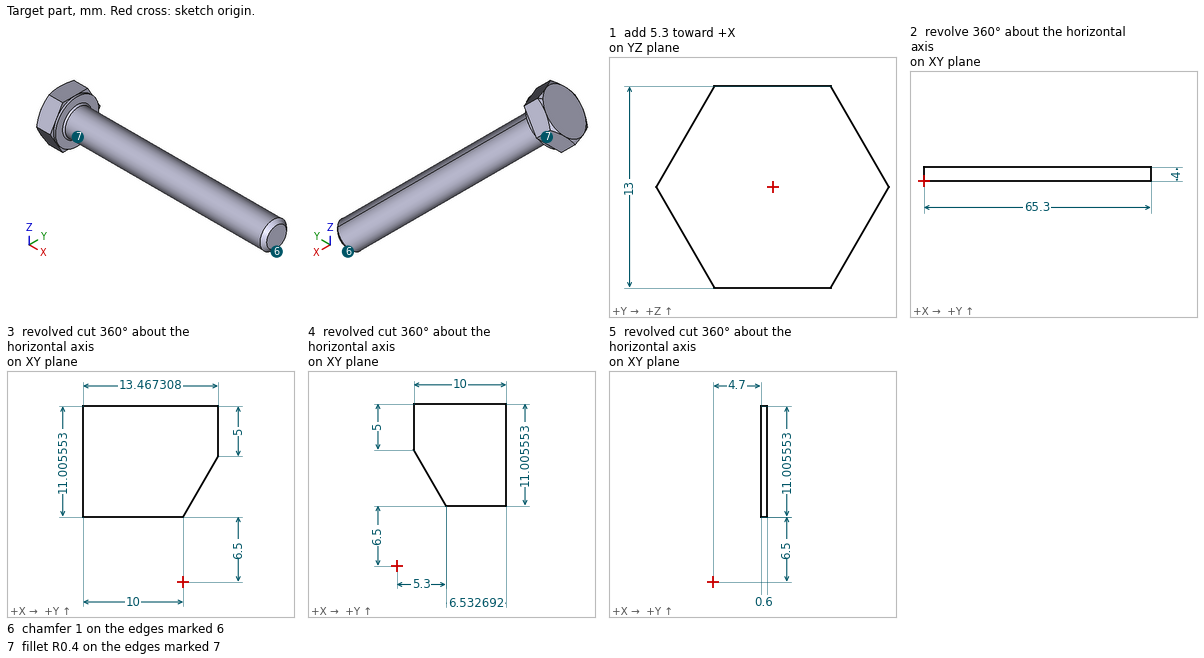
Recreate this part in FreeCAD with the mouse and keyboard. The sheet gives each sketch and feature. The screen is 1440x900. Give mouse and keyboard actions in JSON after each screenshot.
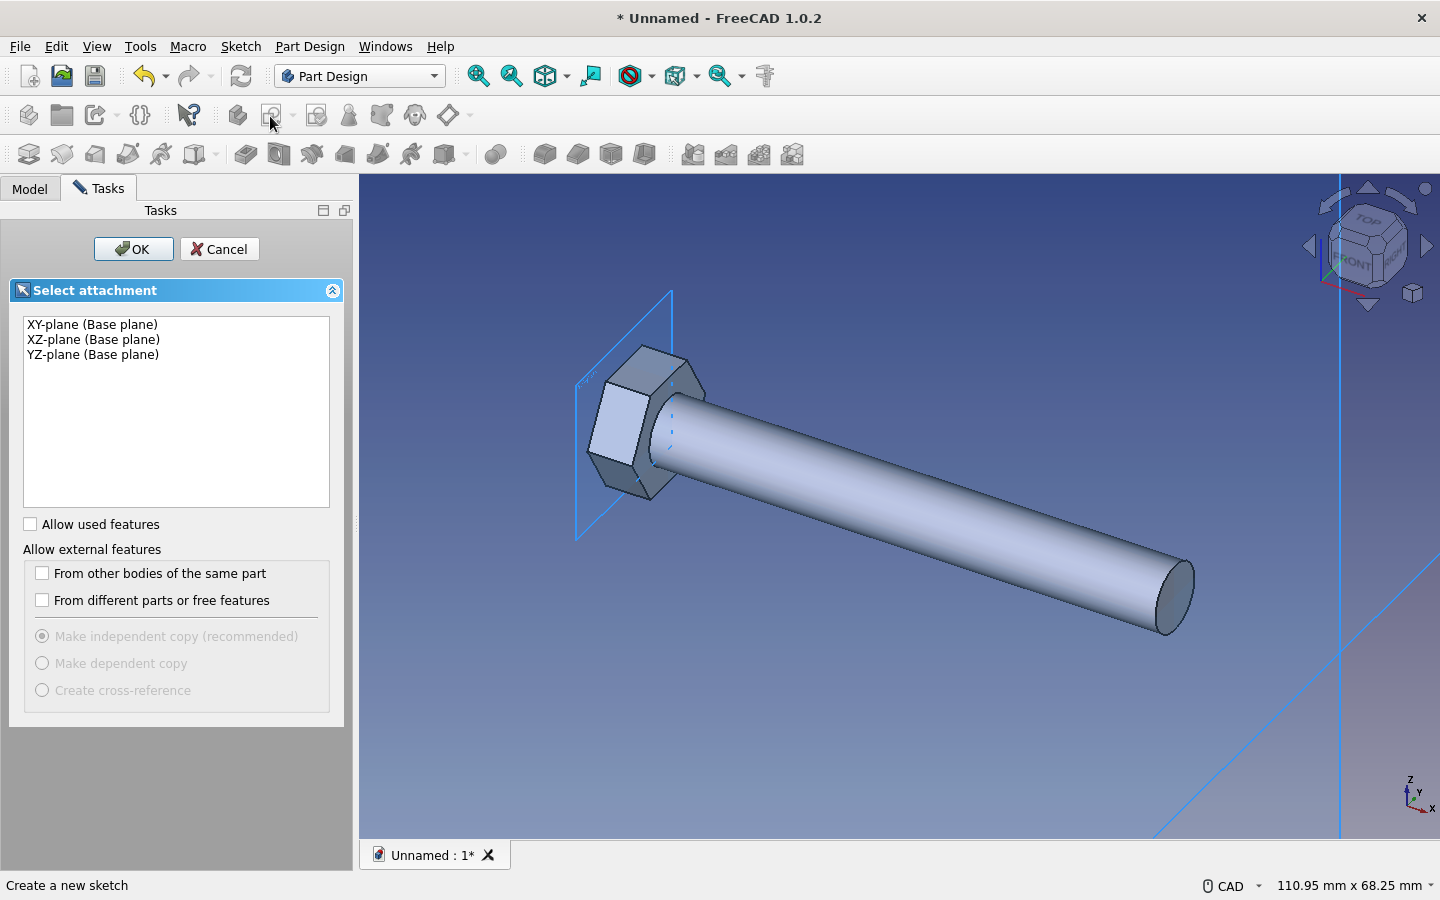
{"action": "left_click", "coordinate": [84, 324]}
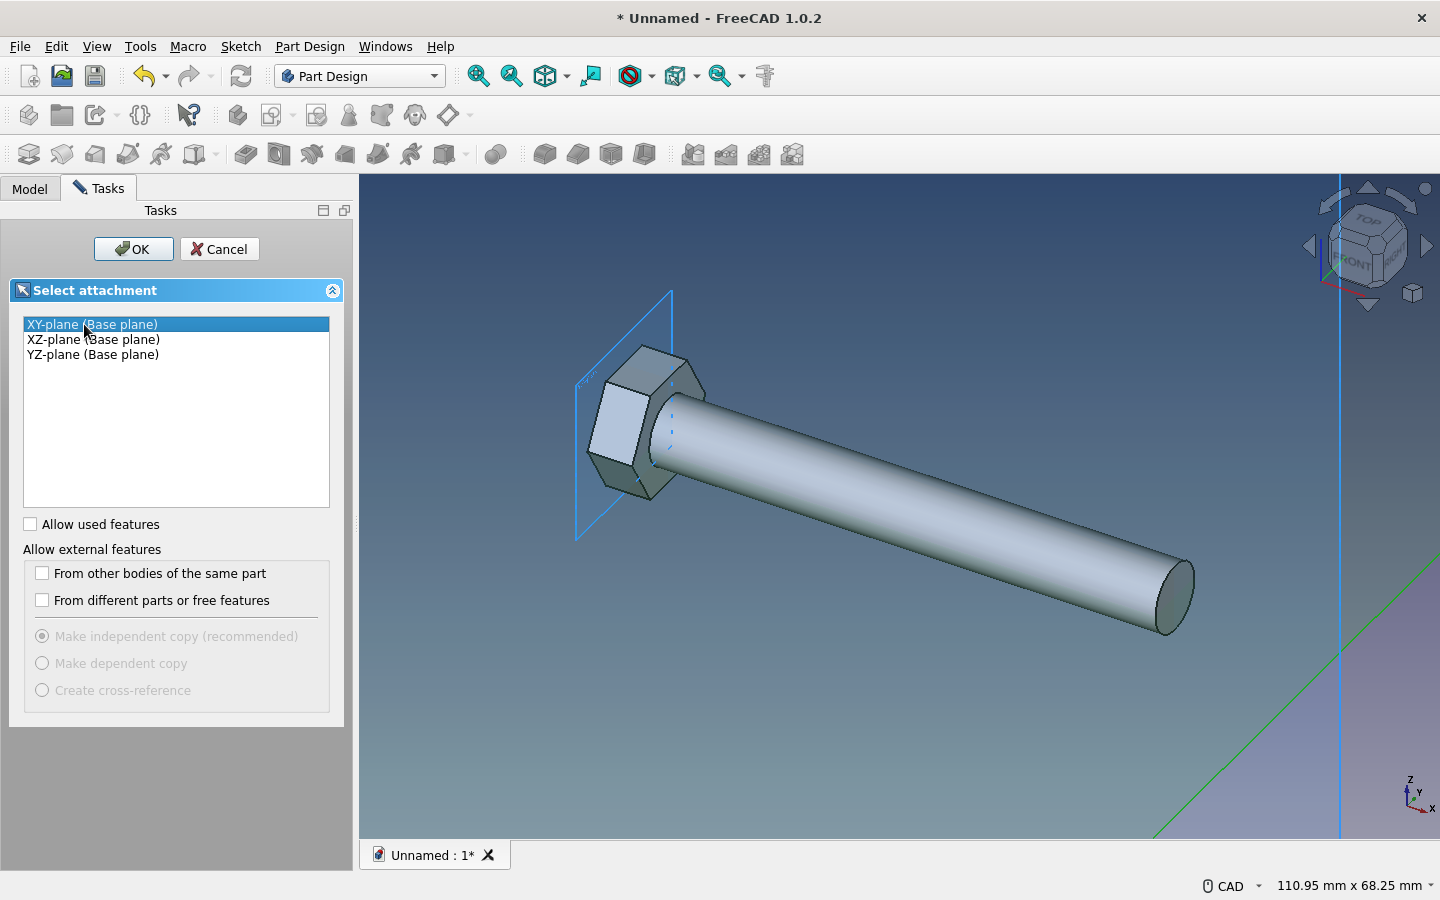
{"action": "left_click", "coordinate": [134, 249]}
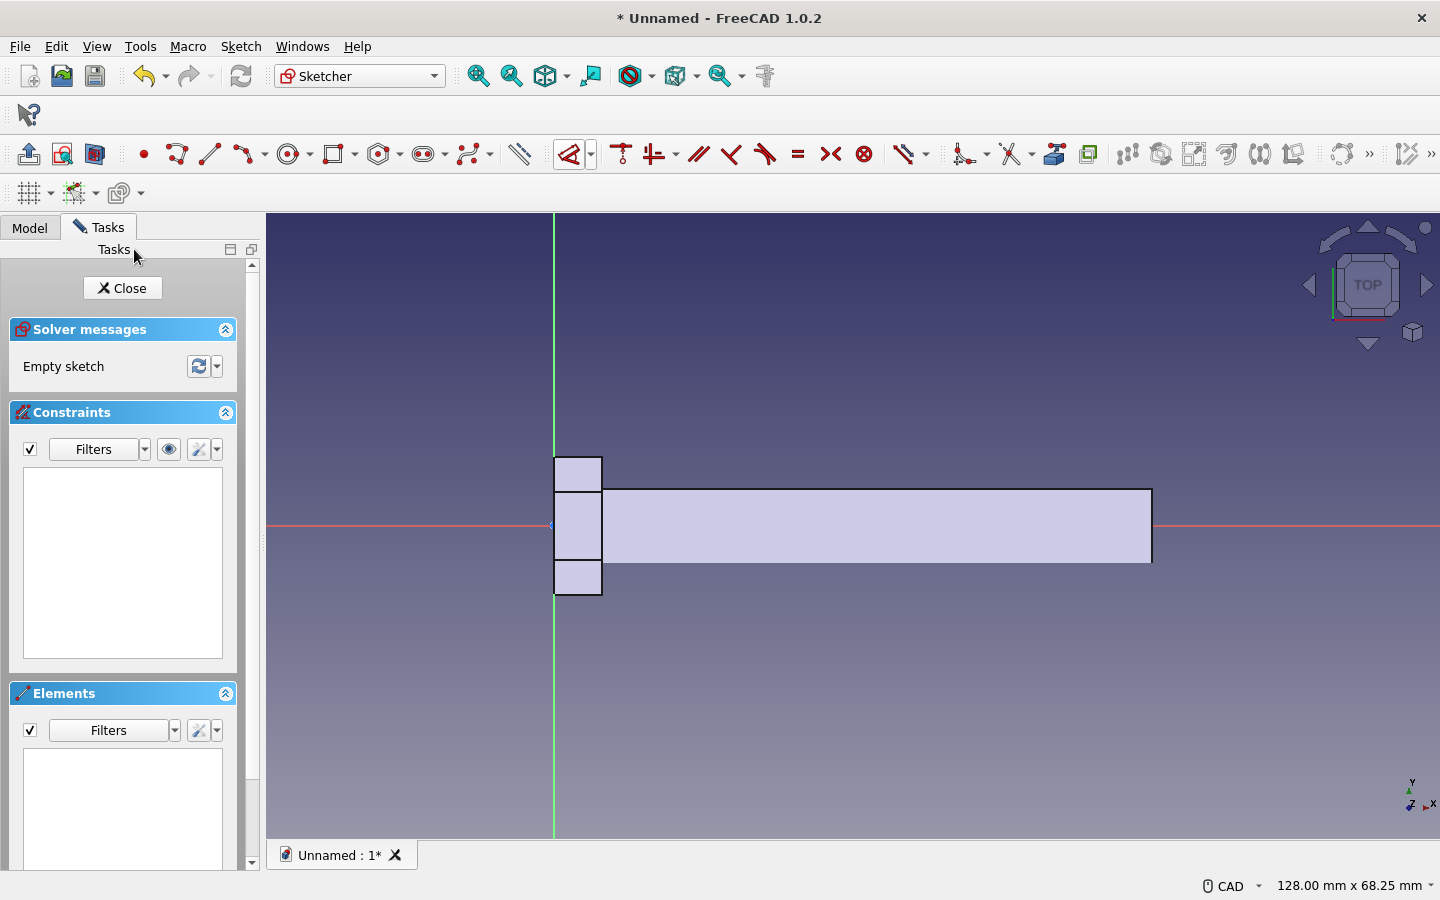
{"action": "left_click", "coordinate": [95, 154]}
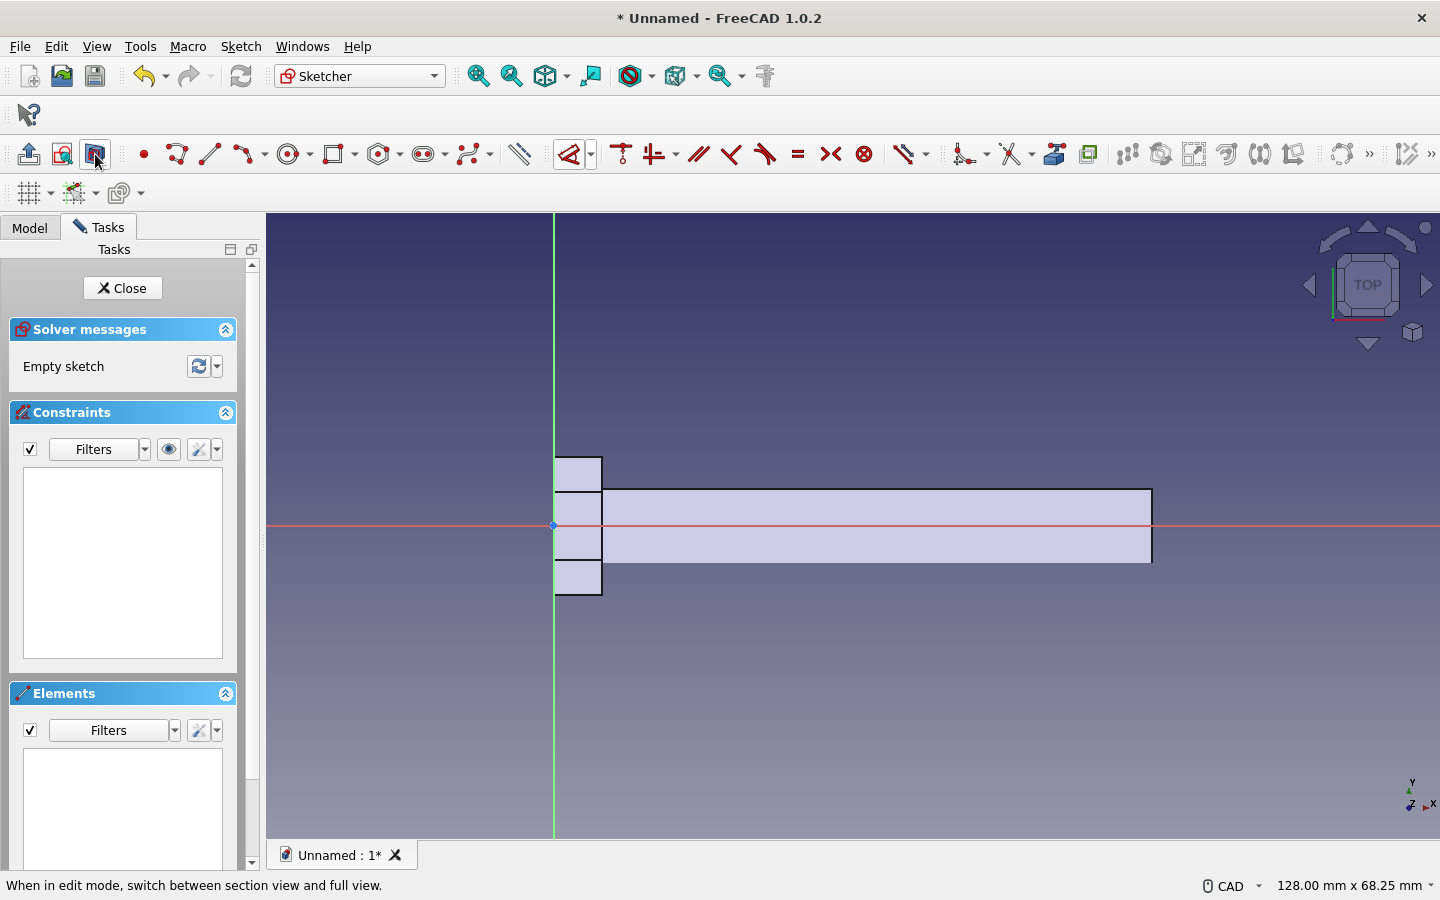
{"action": "scroll", "coordinate": [372, 399], "scroll_direction": "up", "scroll_amount": 5}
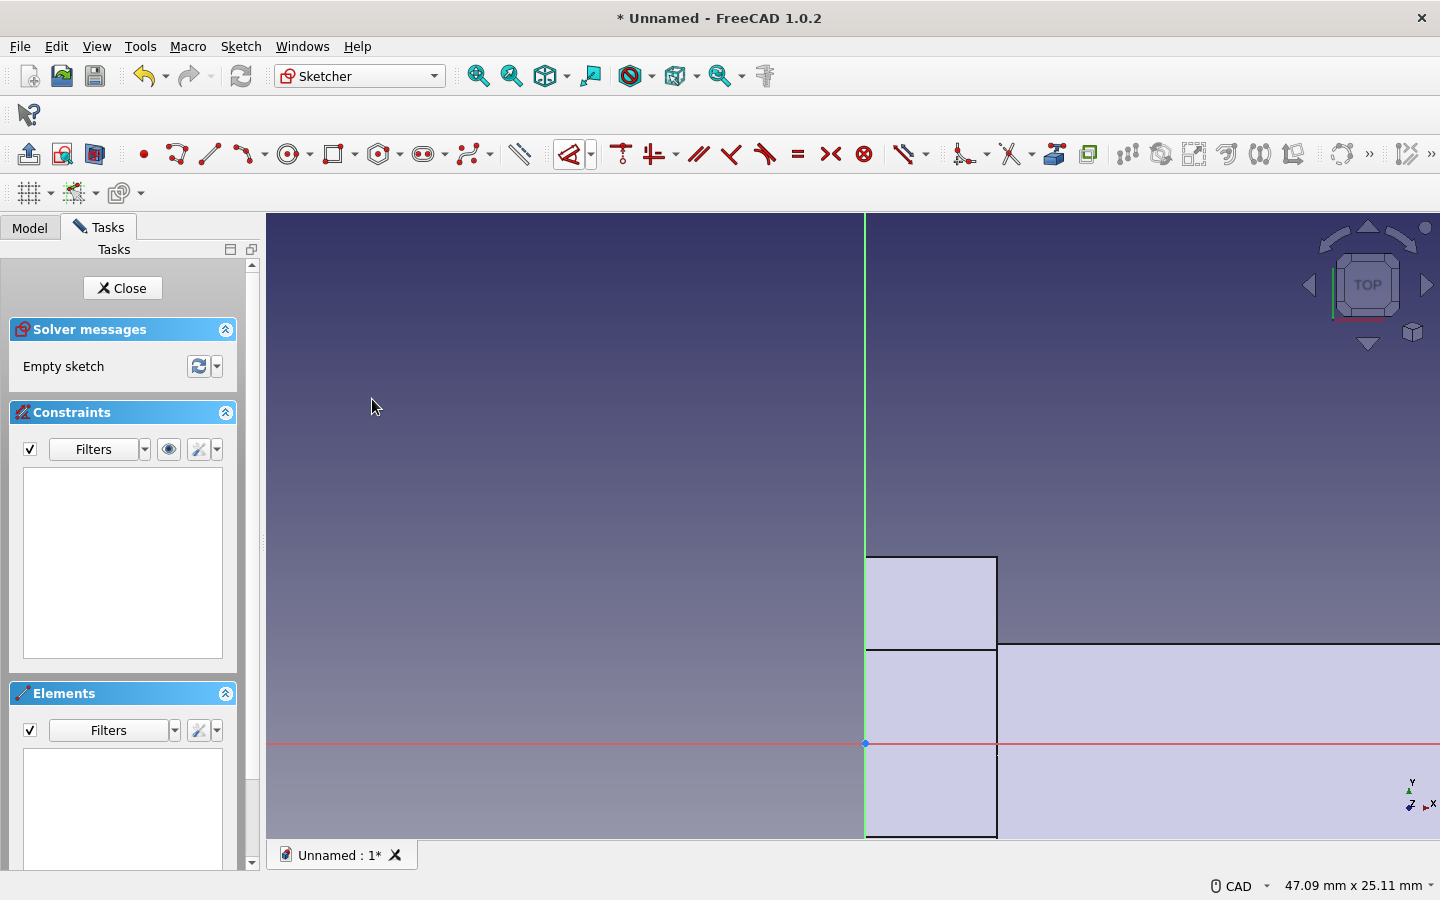
{"action": "left_click", "coordinate": [177, 154]}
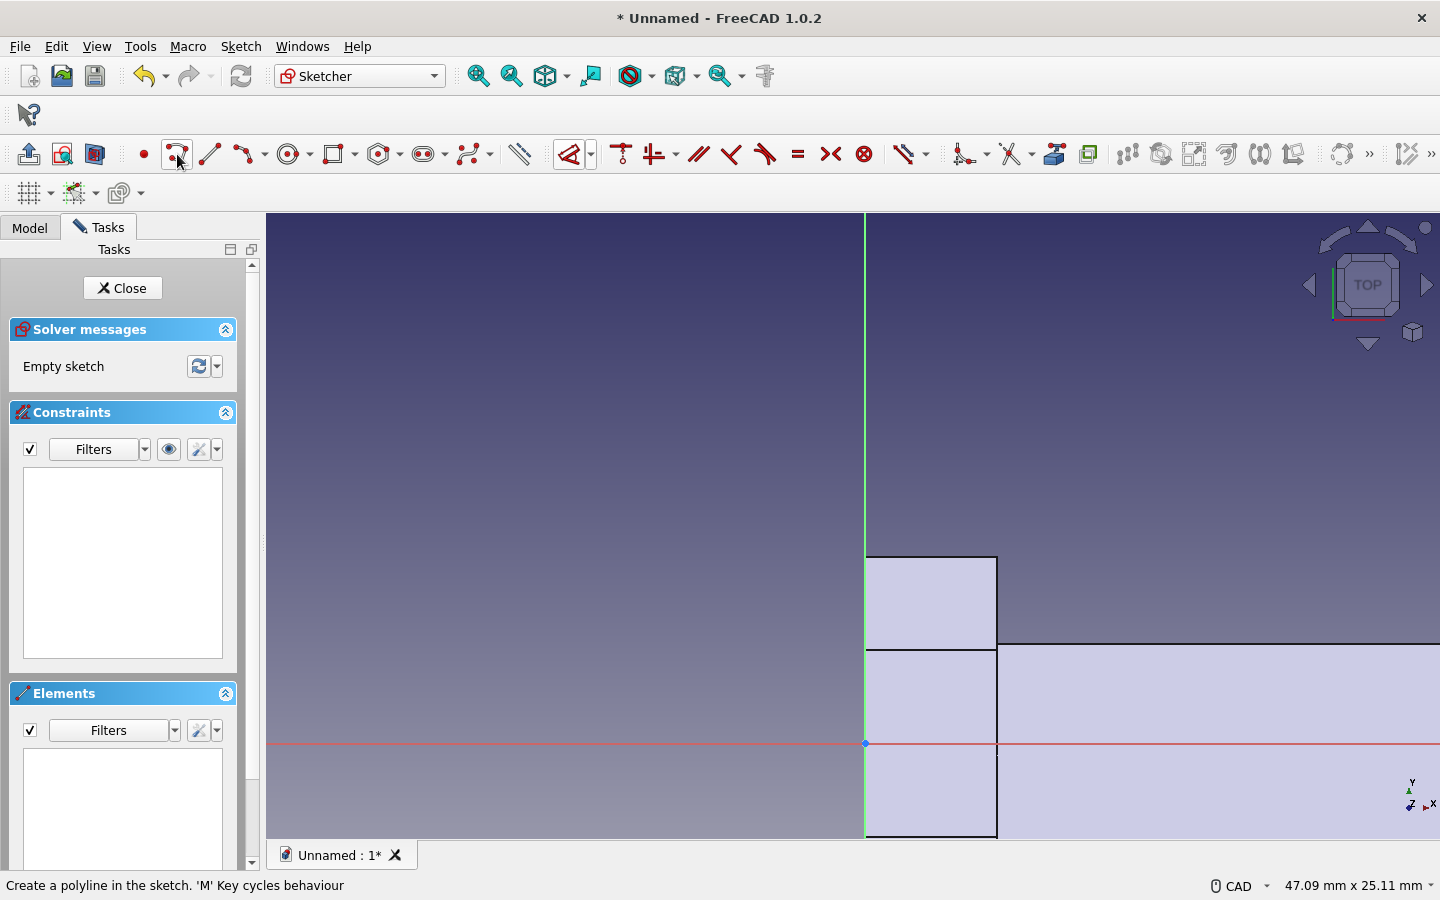
{"action": "left_click", "coordinate": [865, 582]}
{"action": "left_click", "coordinate": [952, 432]}
{"action": "left_click", "coordinate": [952, 307]}
{"action": "left_click", "coordinate": [616, 307]}
{"action": "left_click", "coordinate": [616, 582]}
{"action": "left_click", "coordinate": [865, 583]}
{"action": "key", "text": "Escape"}
{"action": "key", "text": "Escape"}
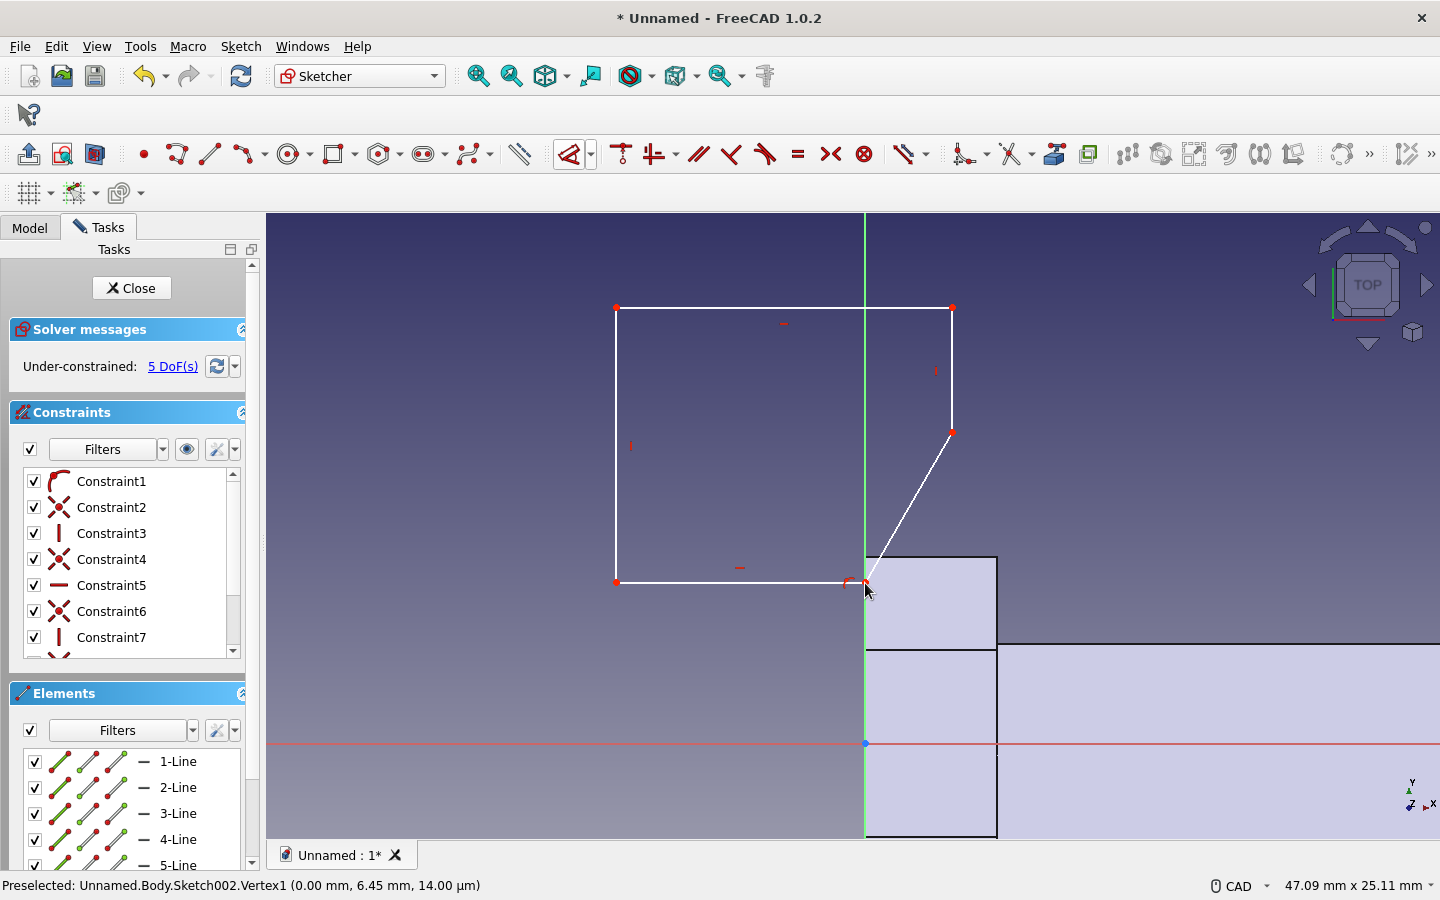
{"action": "left_click", "coordinate": [952, 395]}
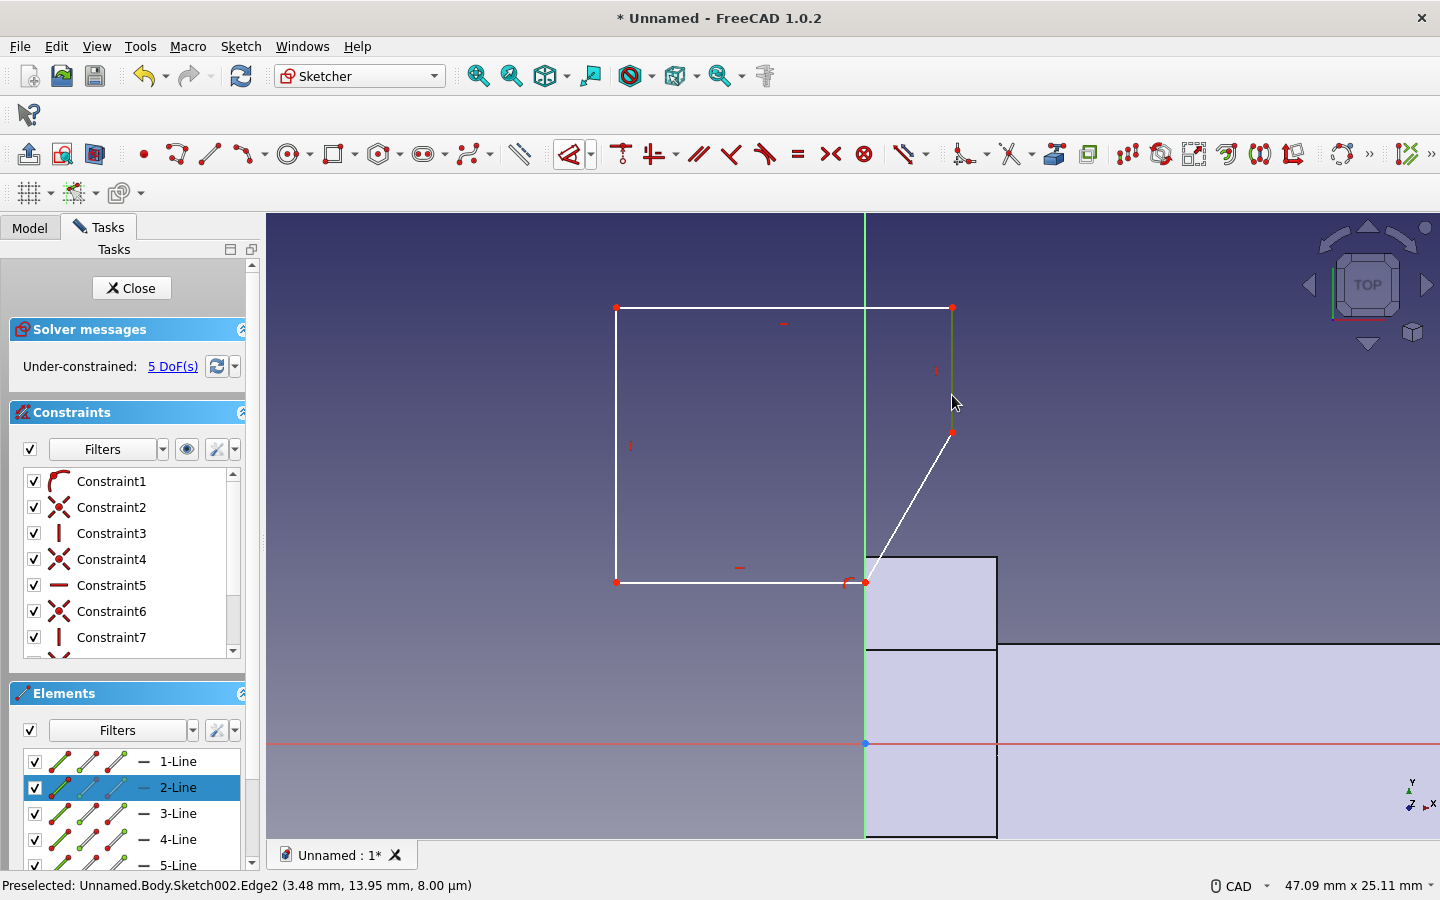
{"action": "key", "text": "i"}